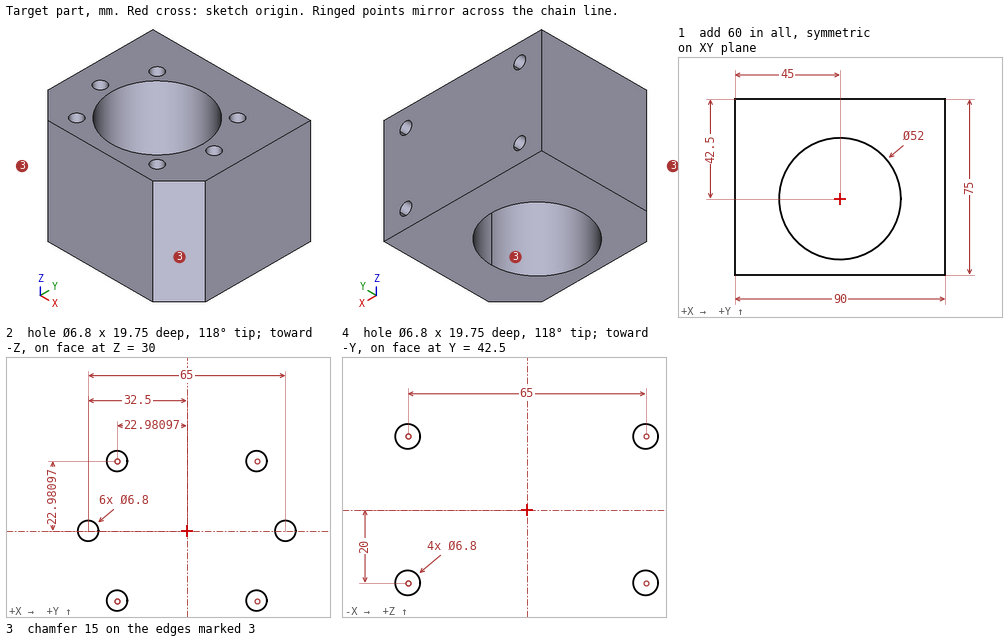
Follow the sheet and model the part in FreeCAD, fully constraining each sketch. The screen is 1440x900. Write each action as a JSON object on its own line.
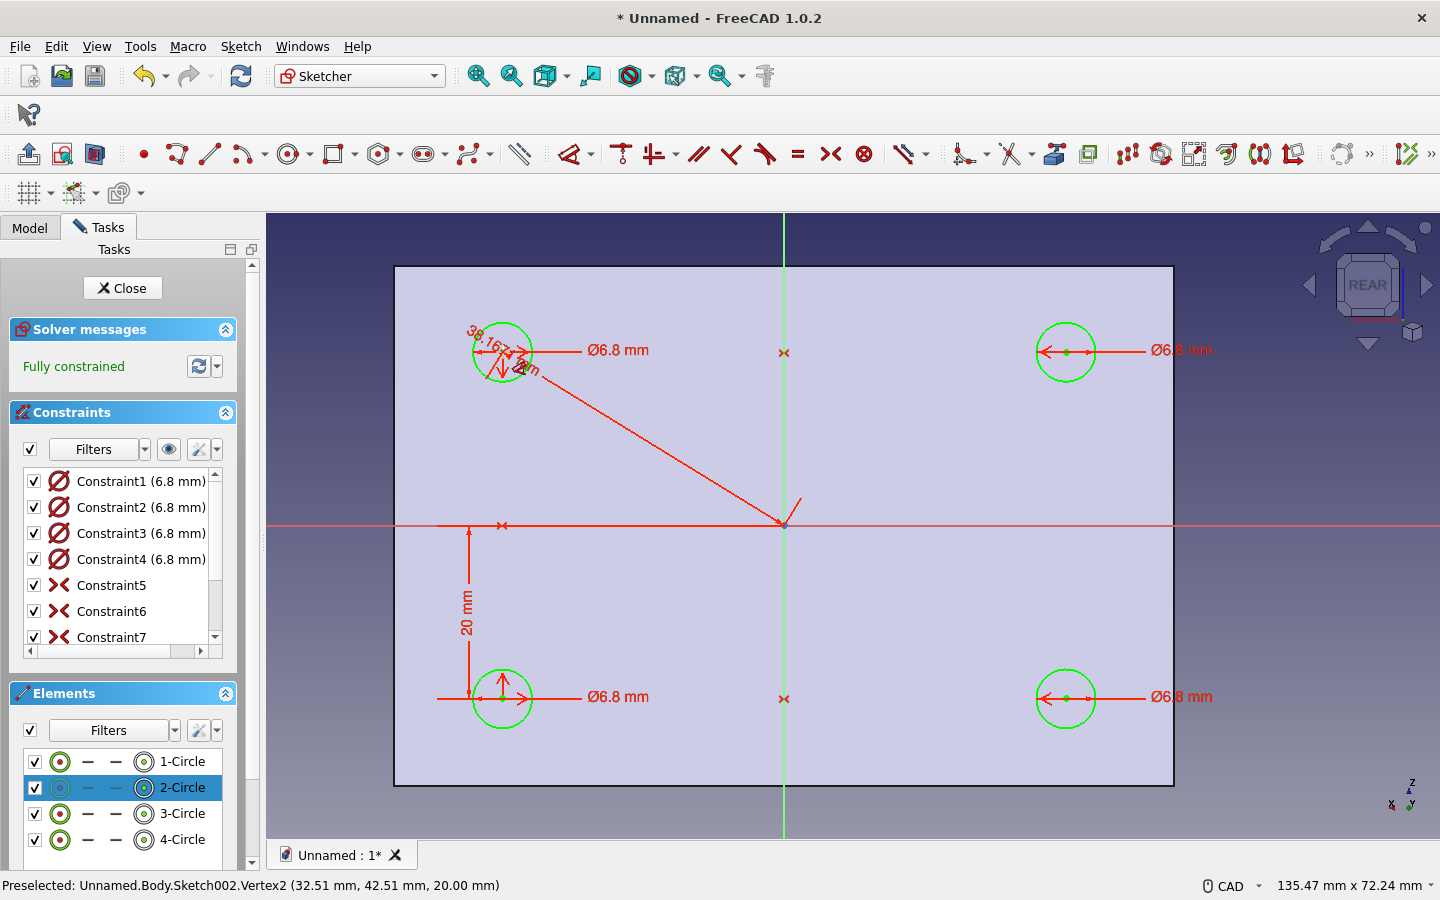
{"action": "left_click", "coordinate": [1066, 352]}
{"action": "left_click", "coordinate": [655, 318]}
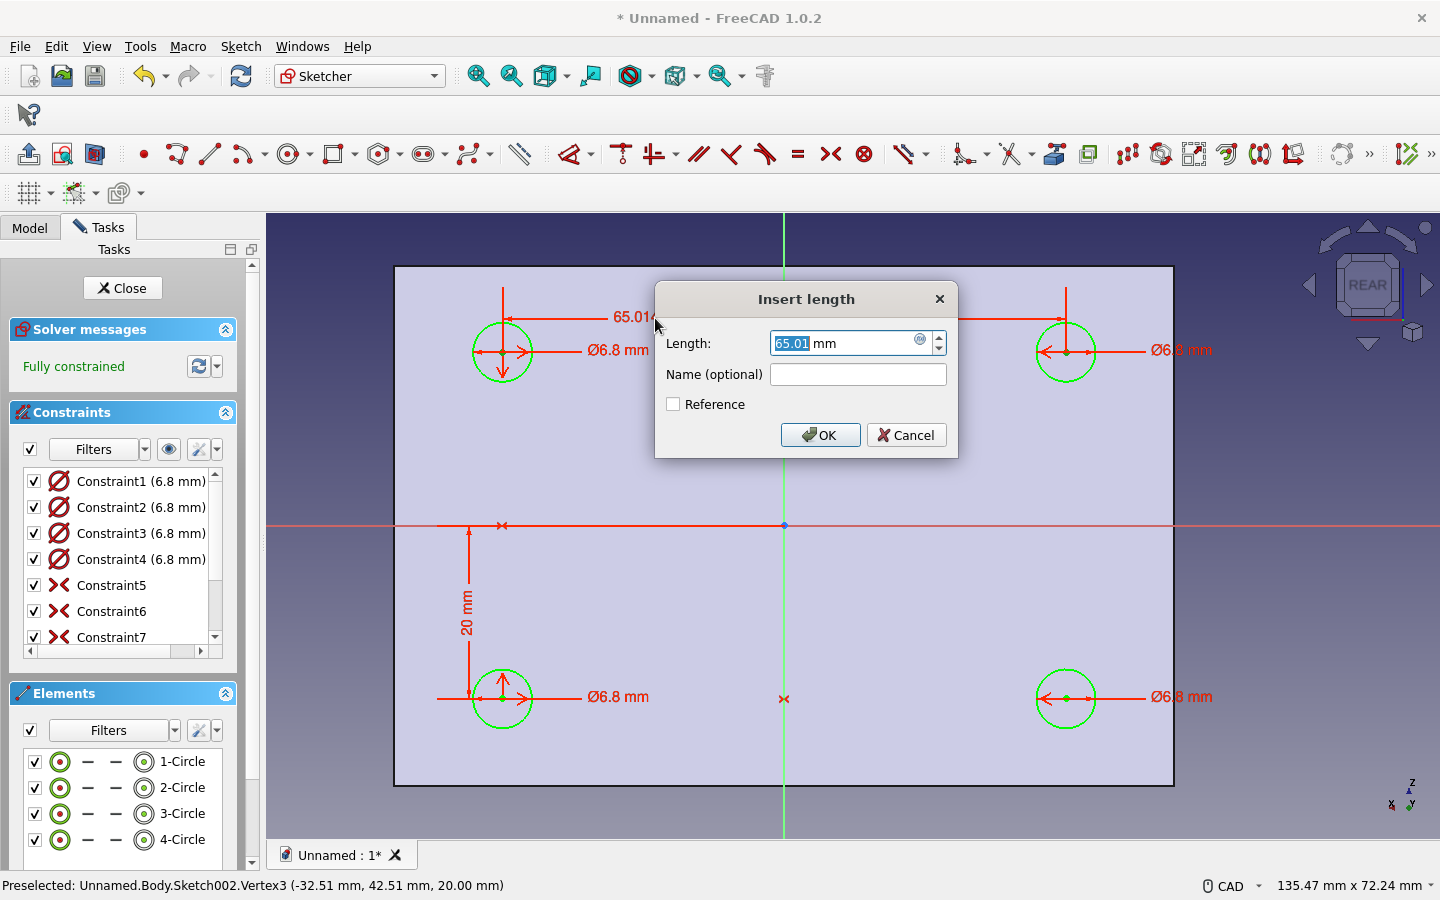
{"action": "type", "text": "65"}
{"action": "key", "text": "Return"}
{"action": "key", "text": "Escape"}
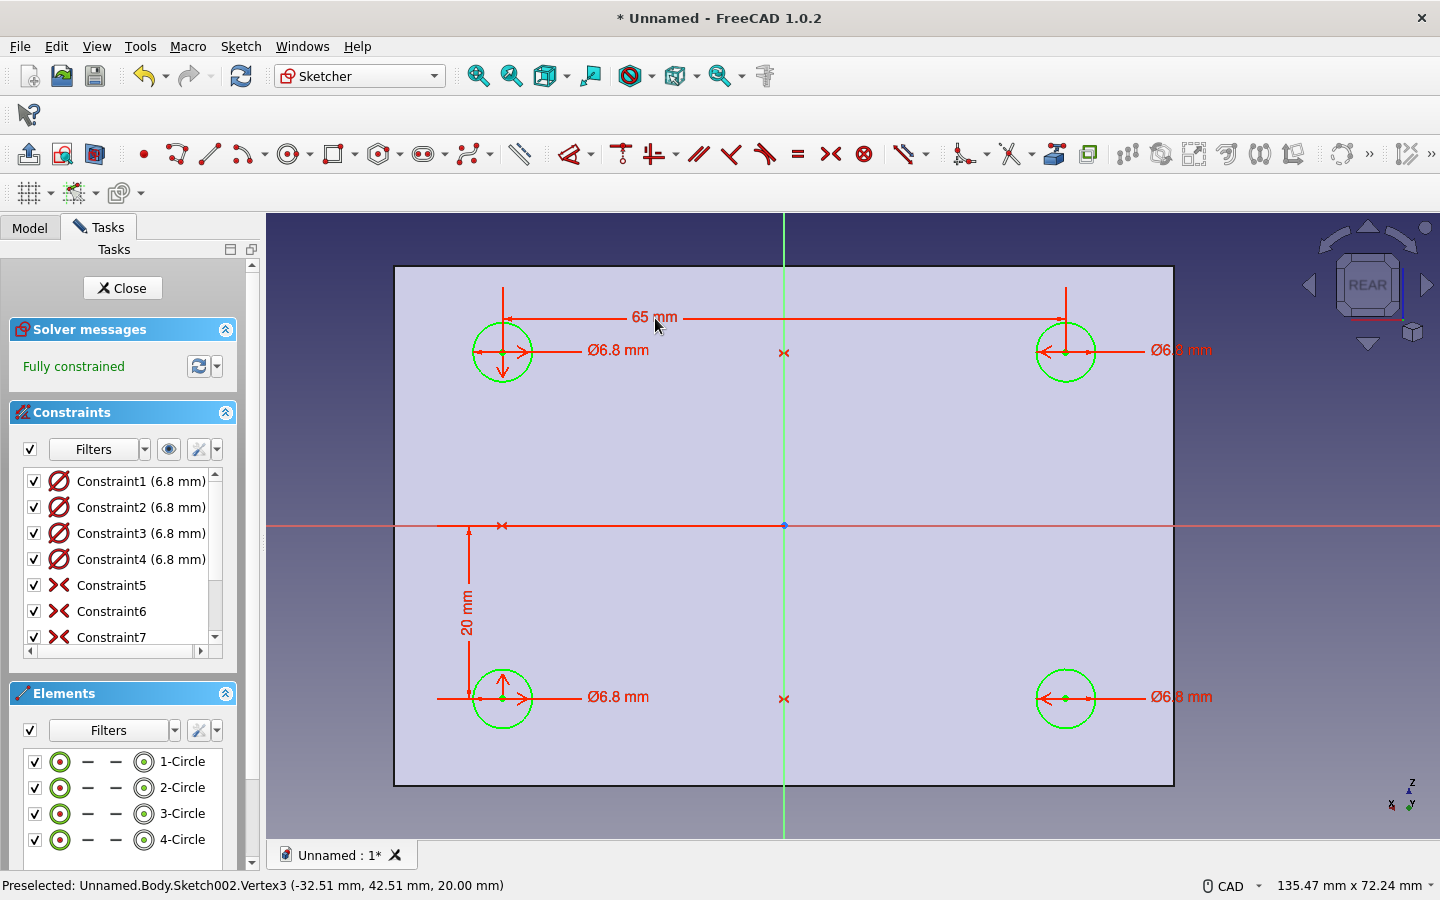
{"action": "left_click", "coordinate": [123, 288]}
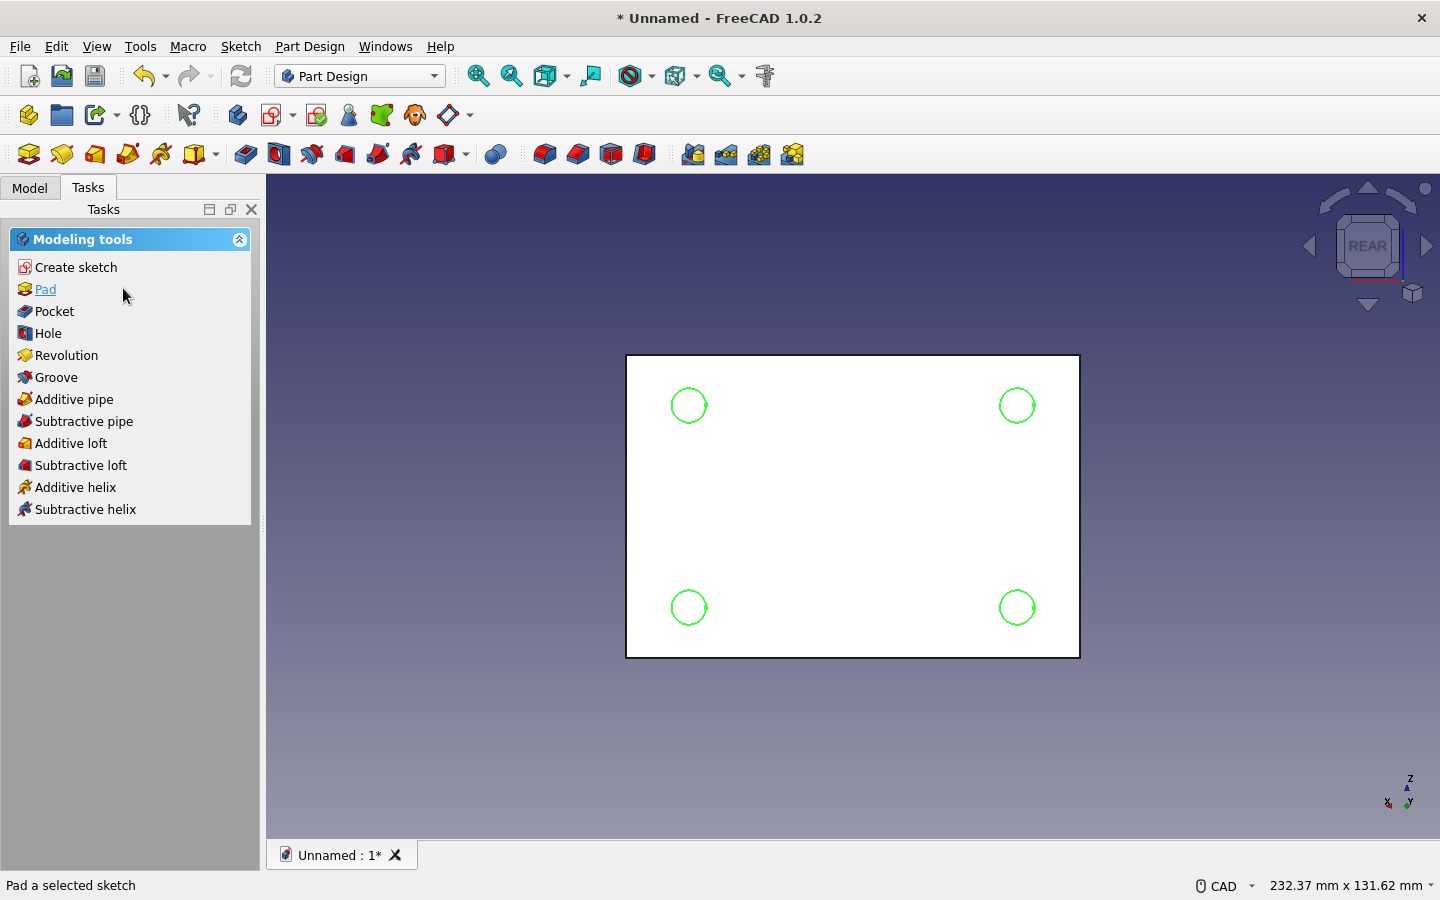
{"action": "left_click", "coordinate": [279, 154]}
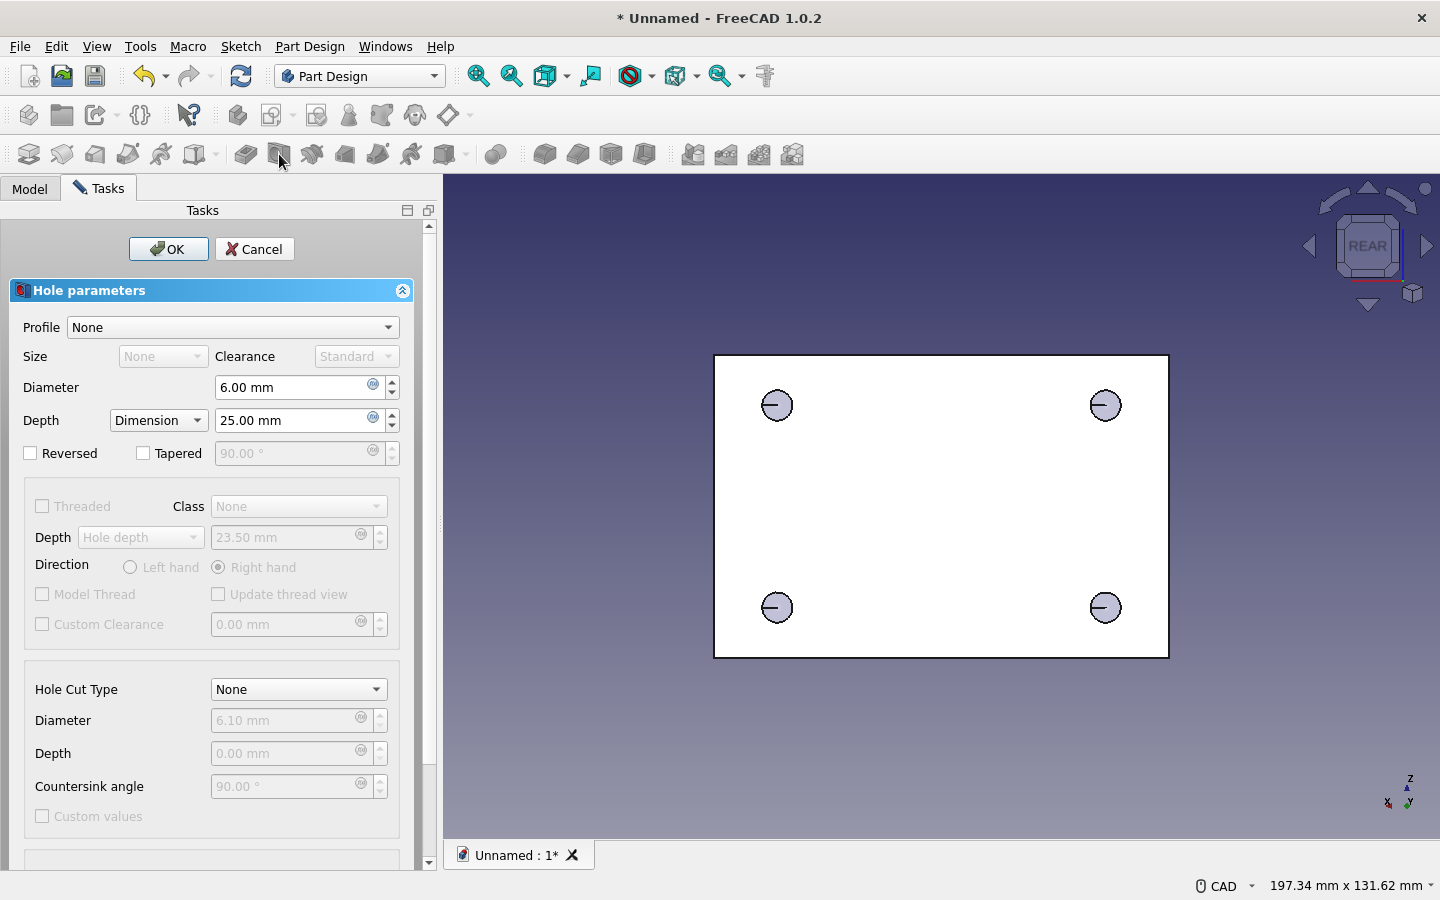
{"action": "triple_click", "coordinate": [300, 388]}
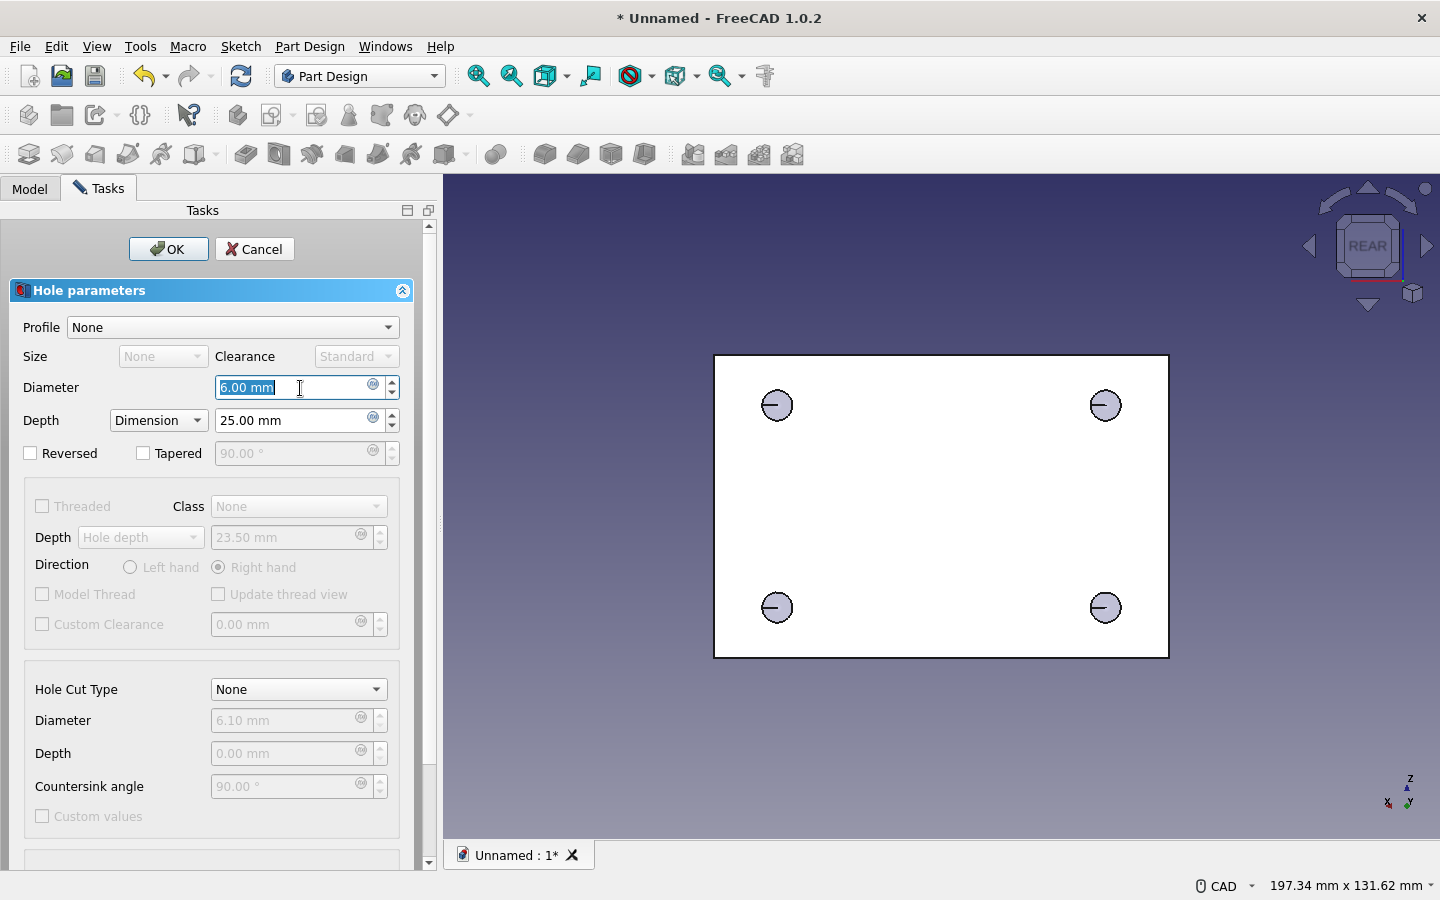
{"action": "type", "text": "6.8"}
{"action": "key", "text": "Tab"}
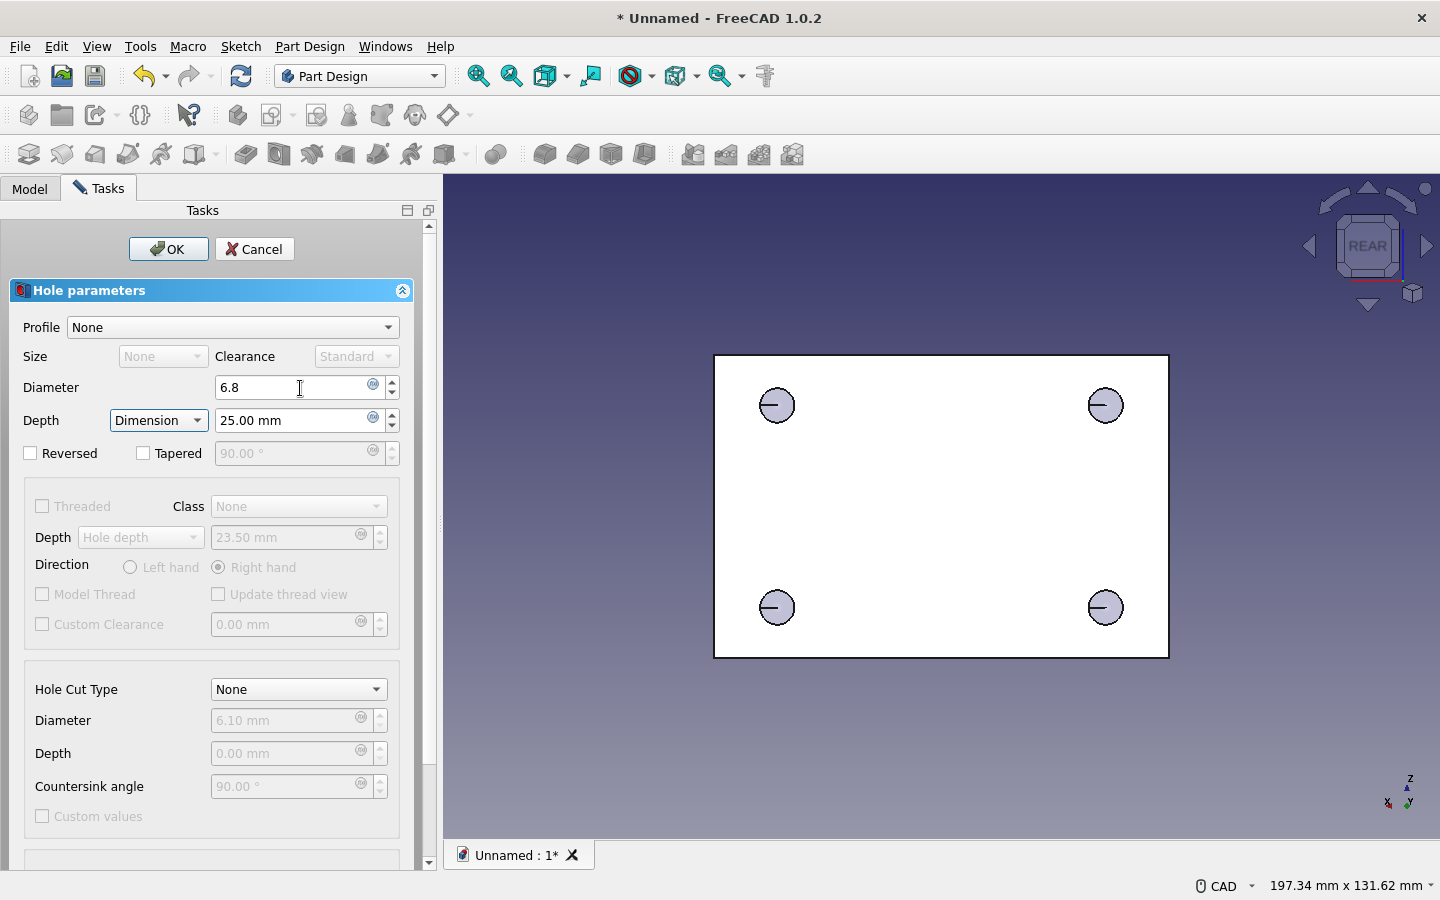
{"action": "triple_click", "coordinate": [300, 420]}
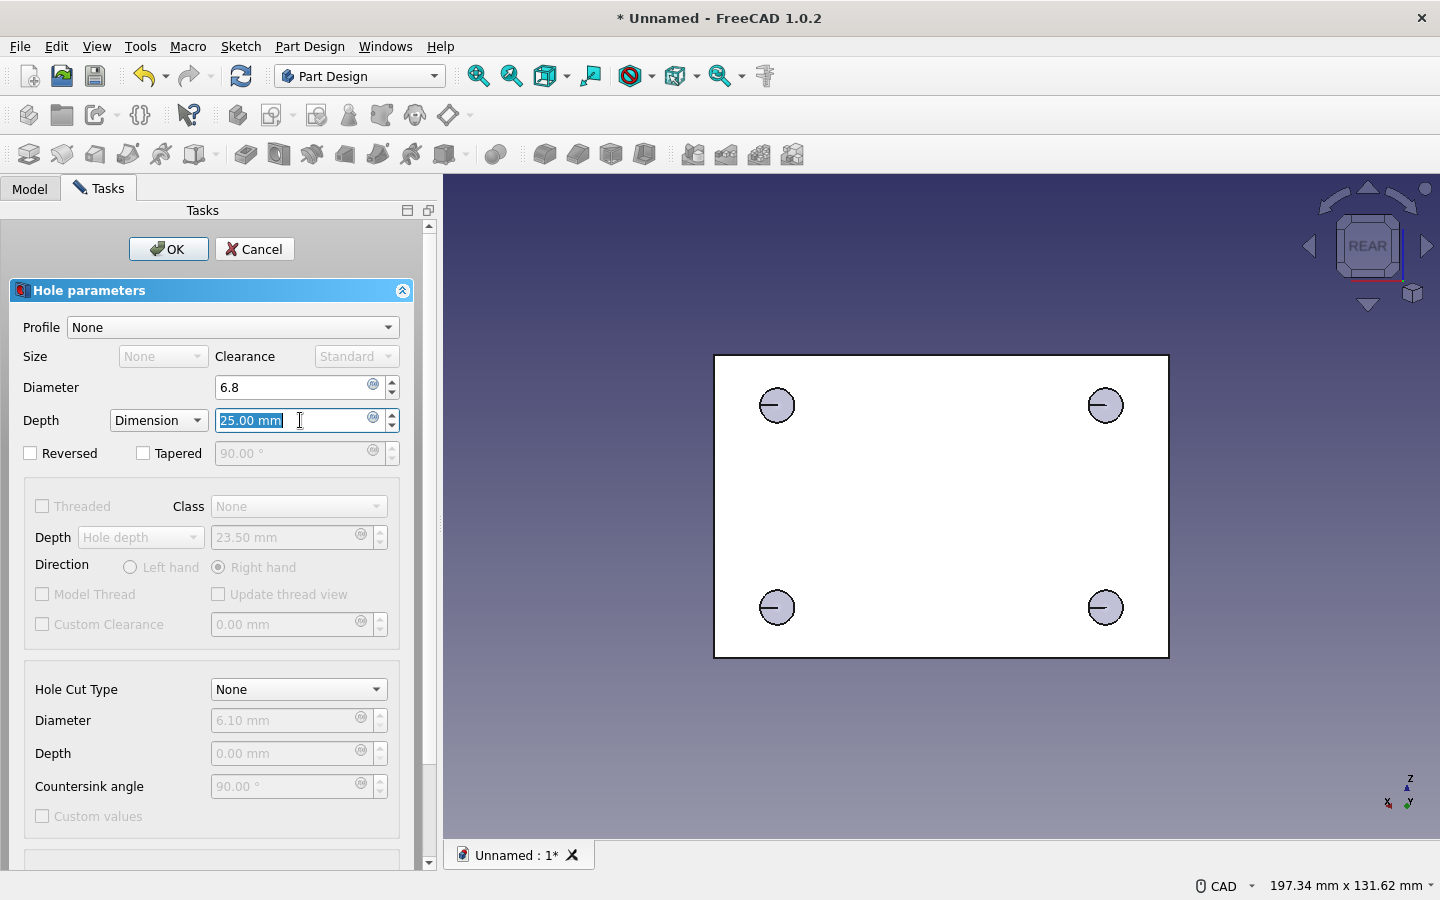
{"action": "type", "text": "19.75"}
{"action": "key", "text": "Tab"}